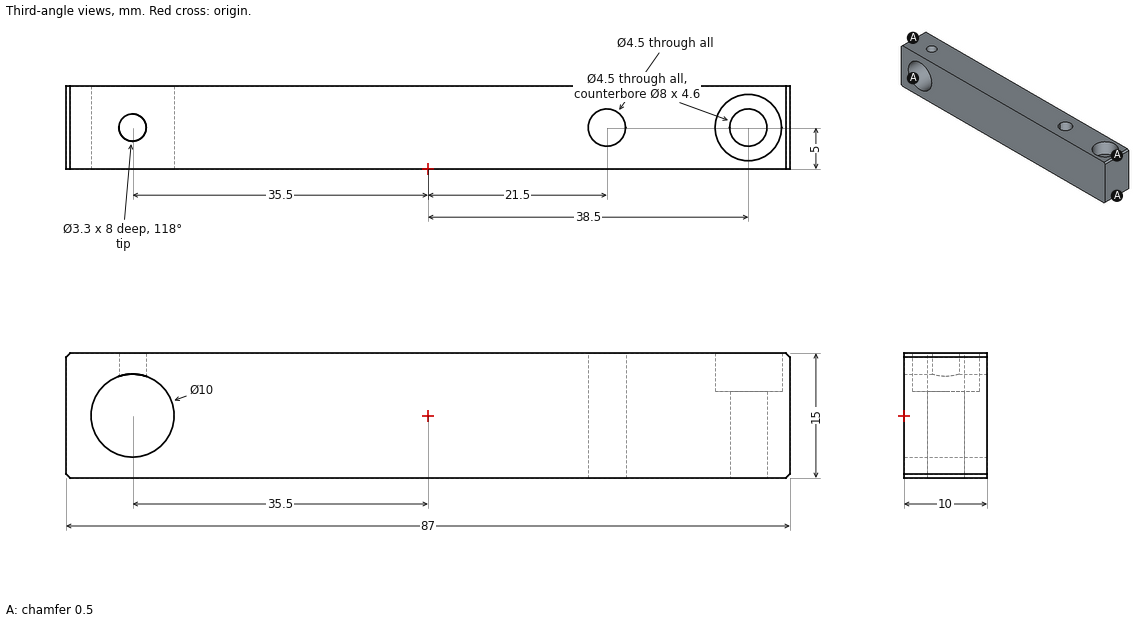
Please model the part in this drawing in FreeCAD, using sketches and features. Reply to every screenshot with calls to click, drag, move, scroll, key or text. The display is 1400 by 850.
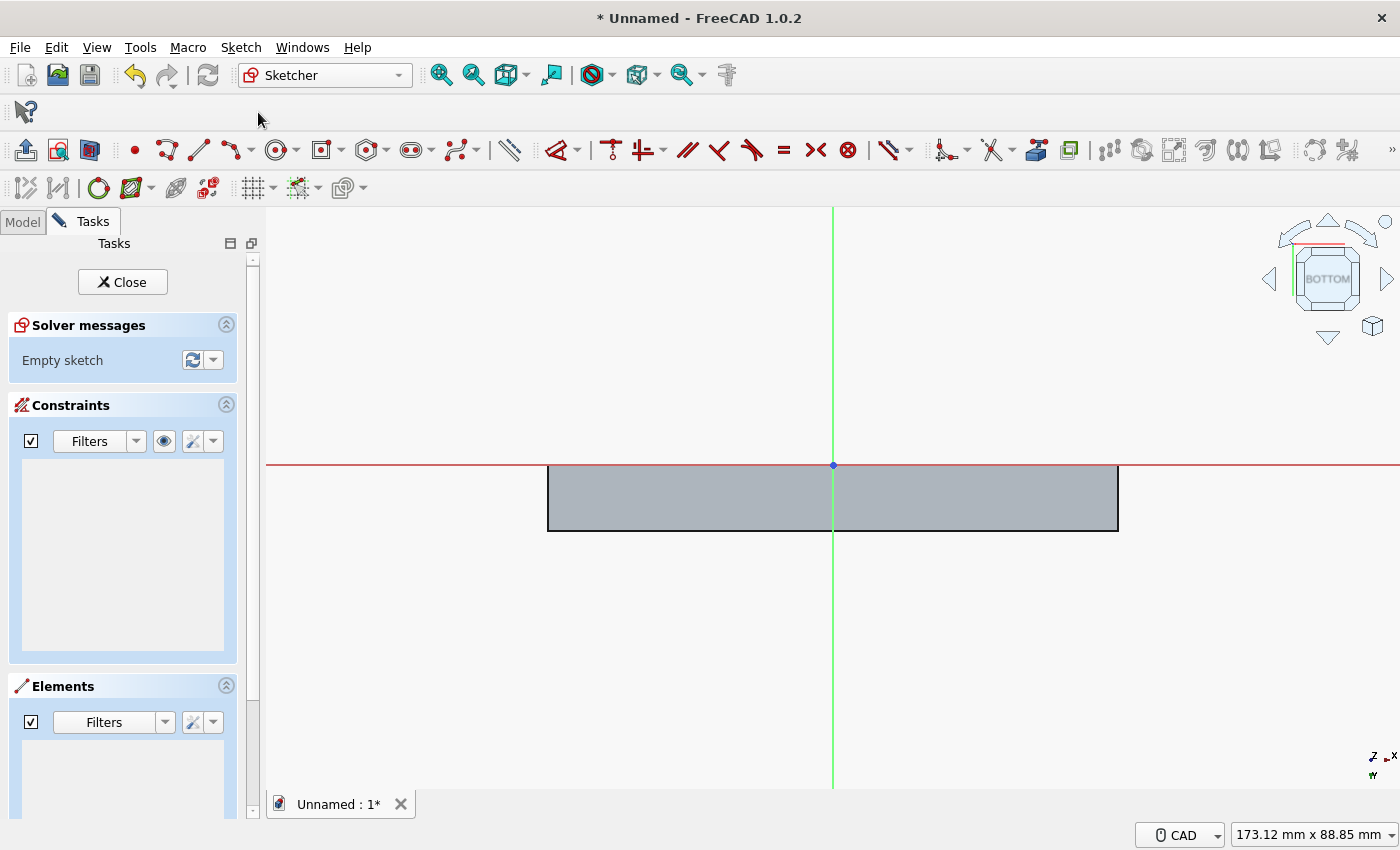
scroll(991, 498, up, 13)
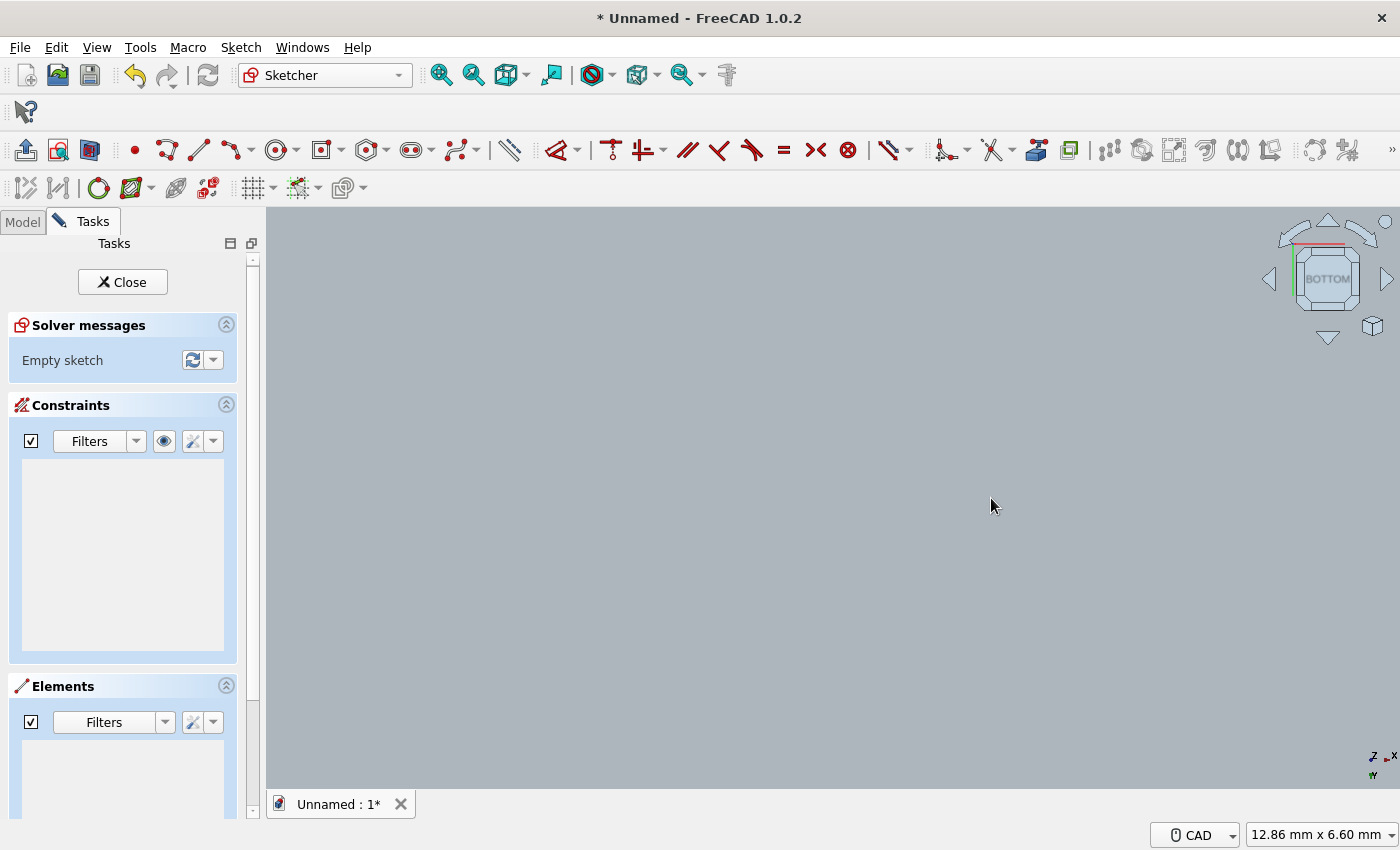
click(276, 150)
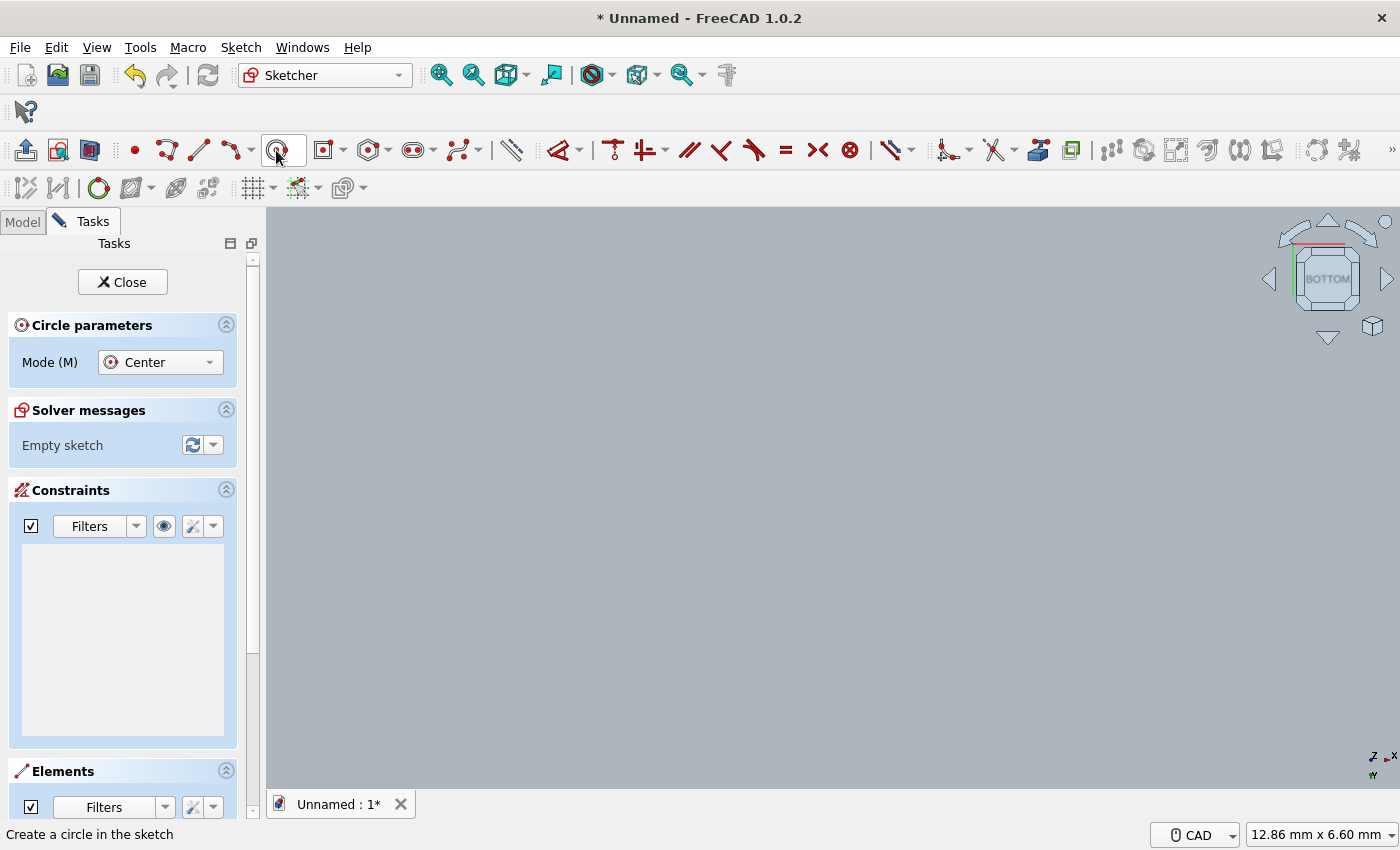
click(752, 492)
click(892, 351)
key(Escape)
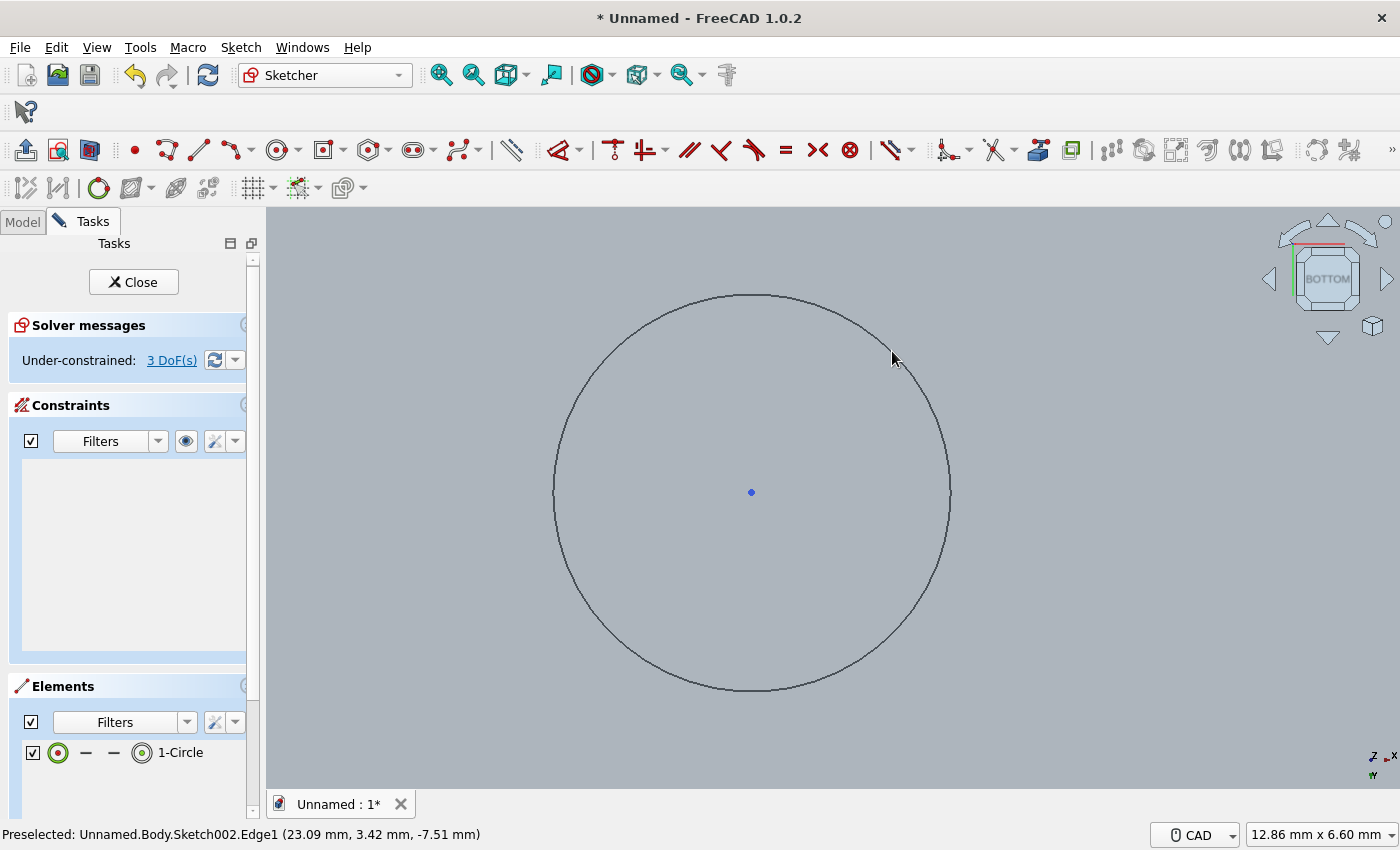
click(558, 150)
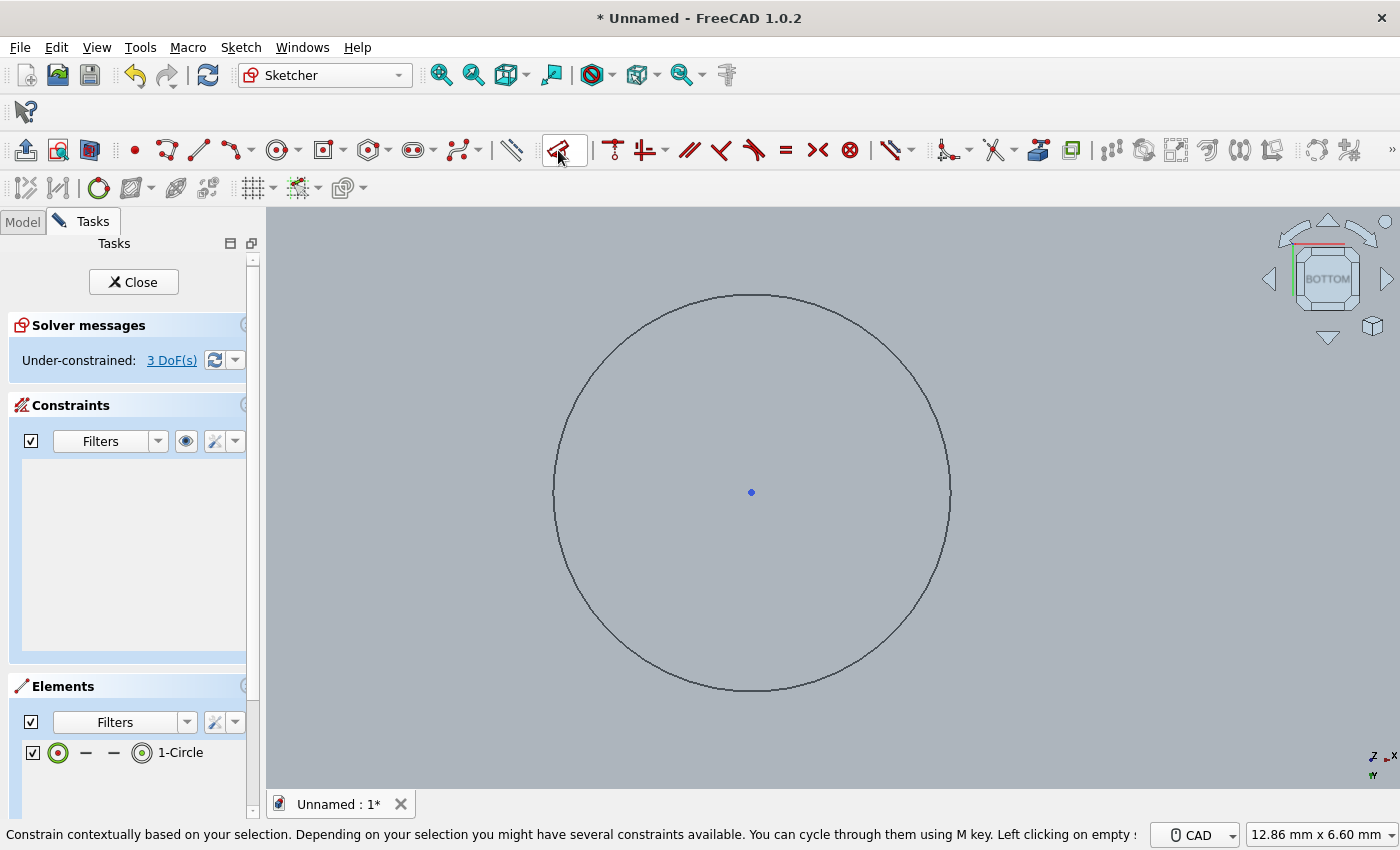
click(892, 352)
click(915, 329)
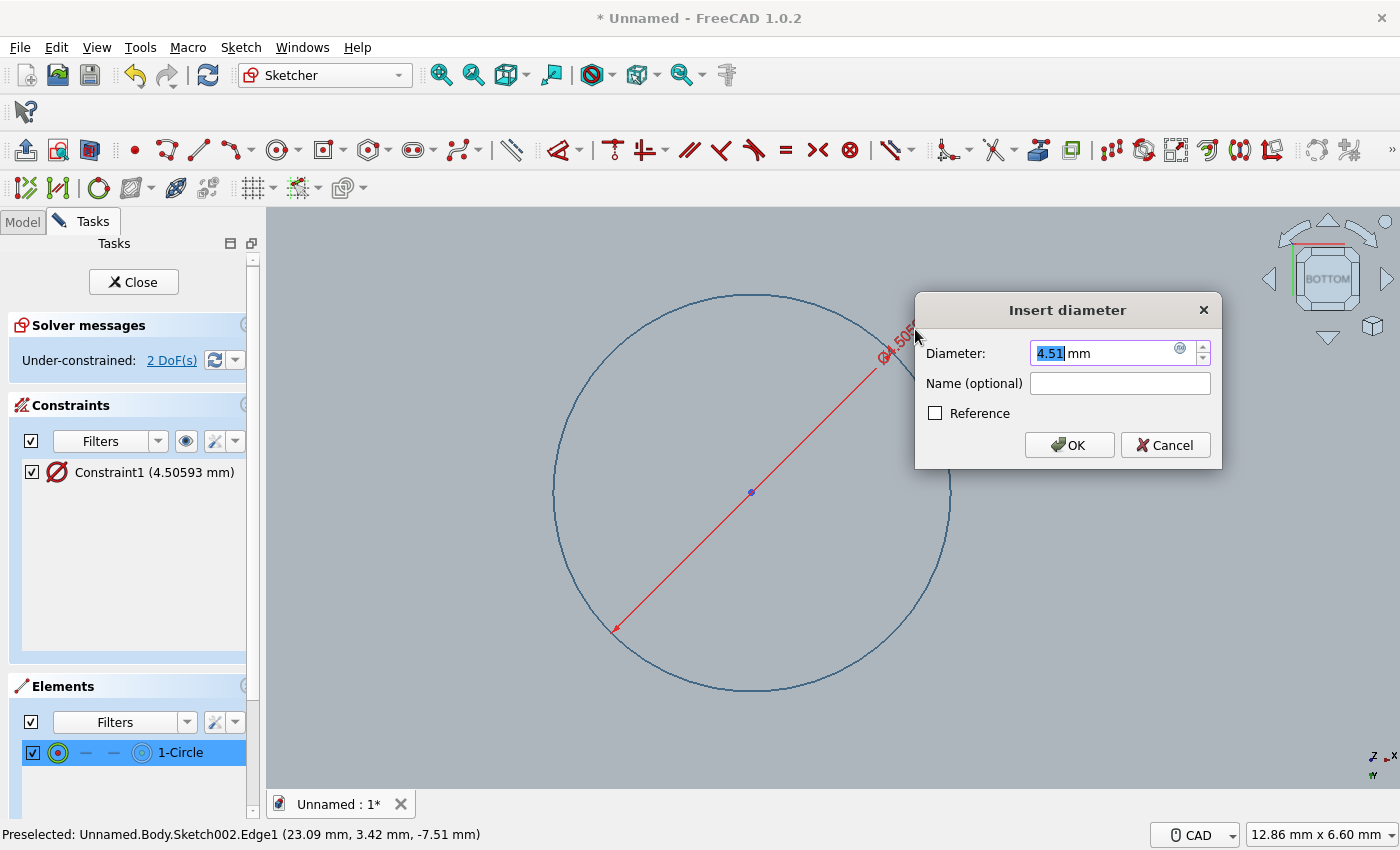
text(4.5)
key(Return)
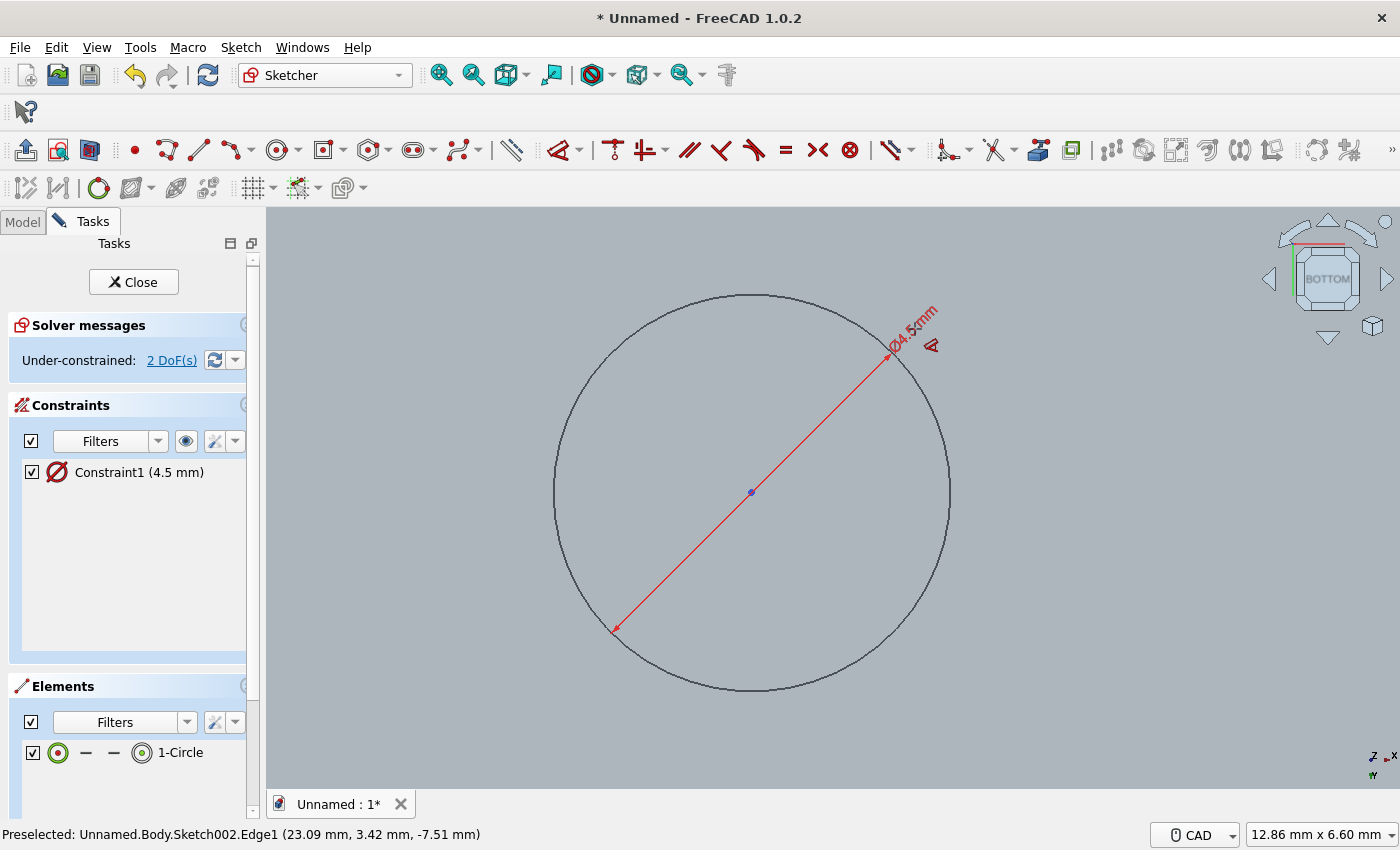
click(752, 493)
click(786, 364)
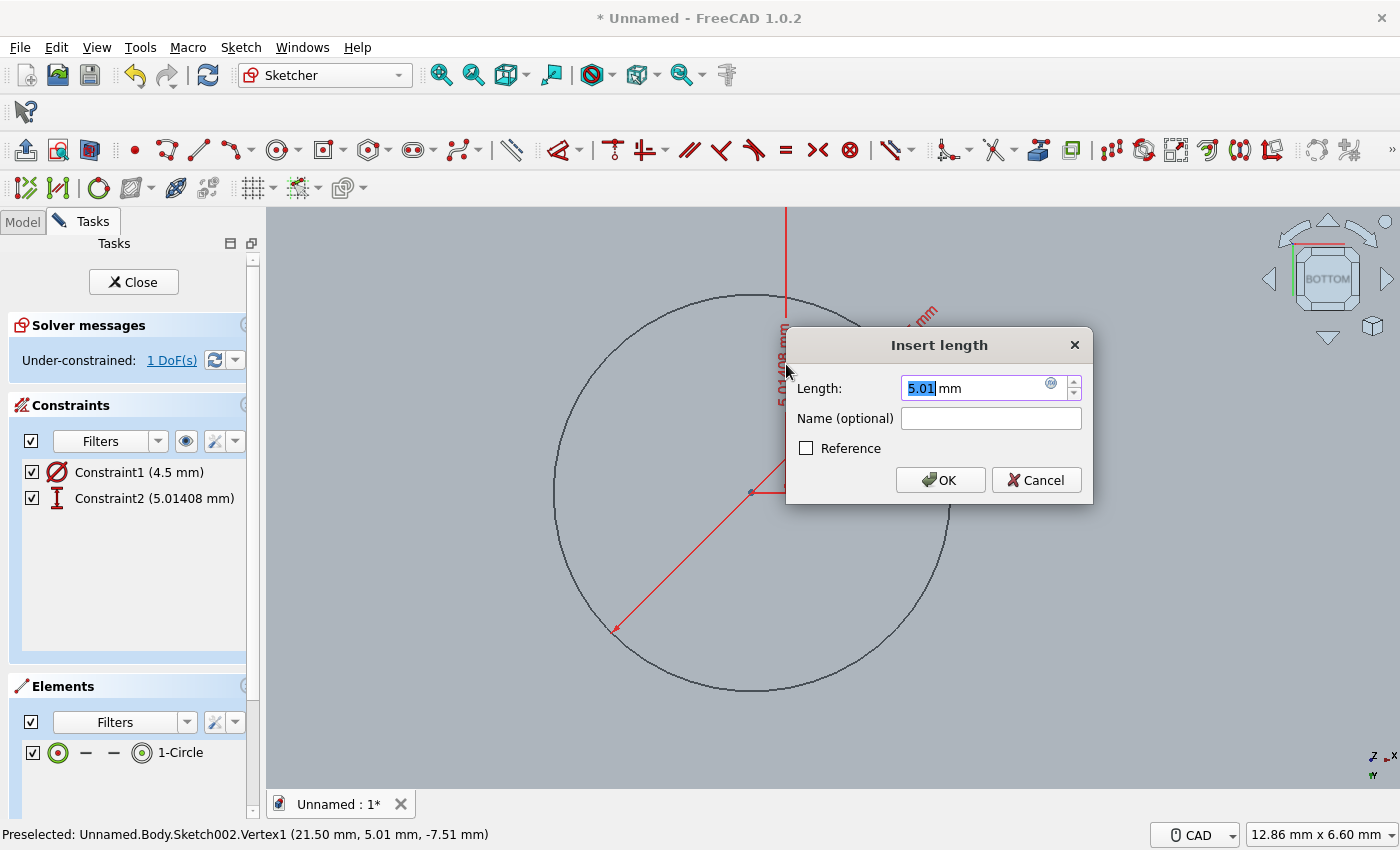
text(5)
key(Return)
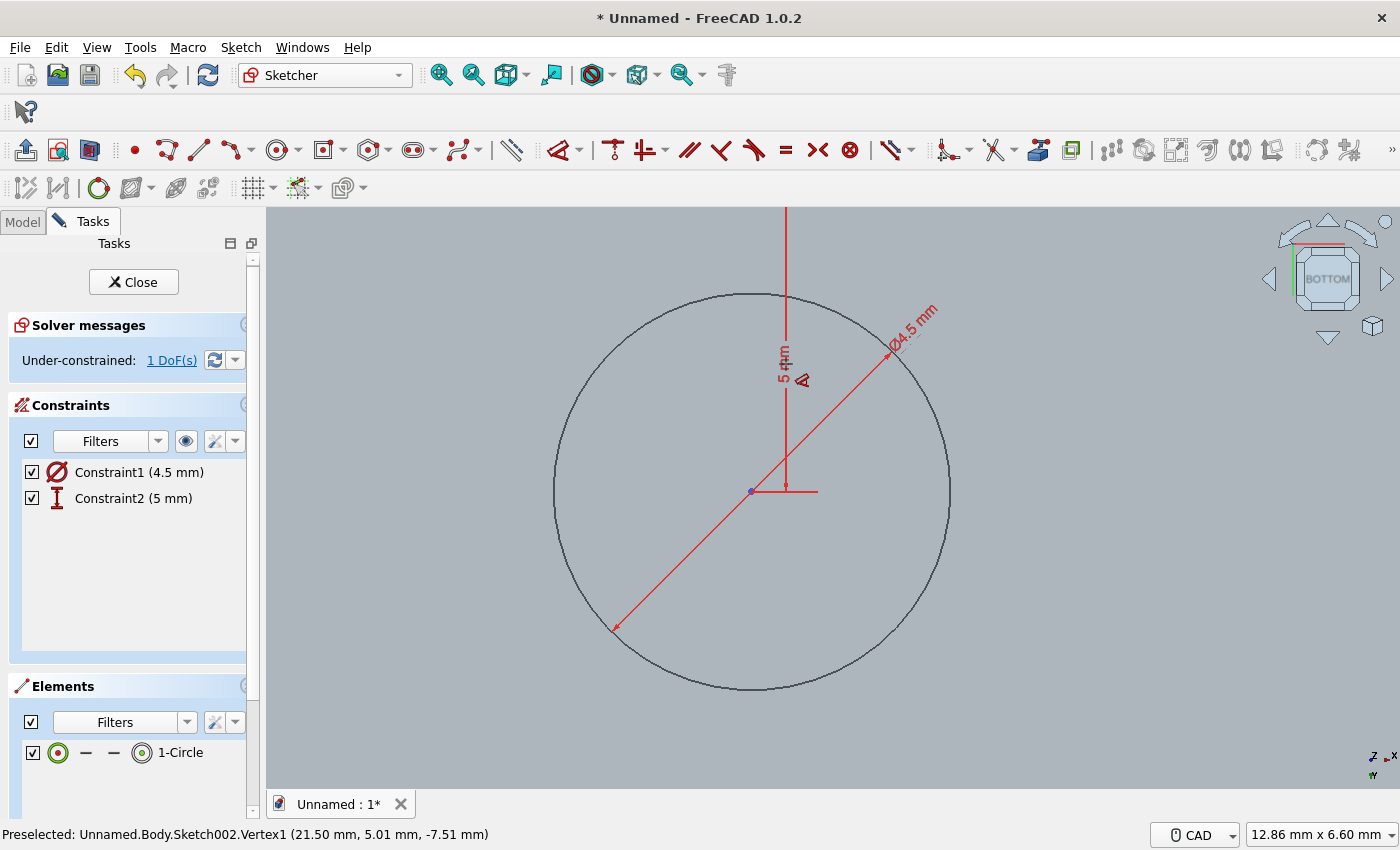
click(752, 492)
click(523, 526)